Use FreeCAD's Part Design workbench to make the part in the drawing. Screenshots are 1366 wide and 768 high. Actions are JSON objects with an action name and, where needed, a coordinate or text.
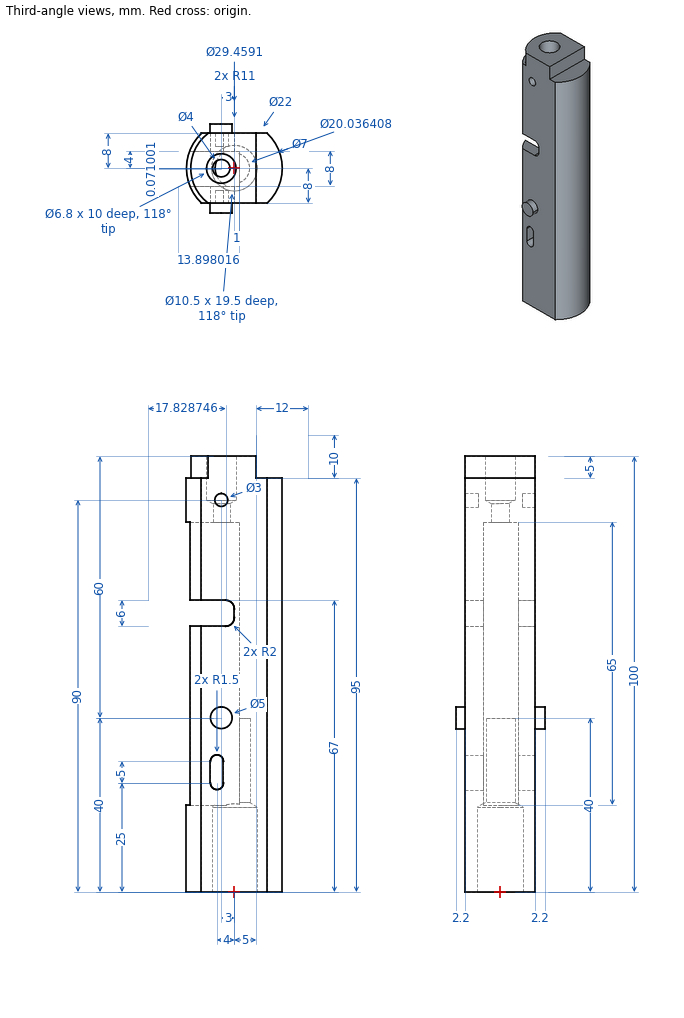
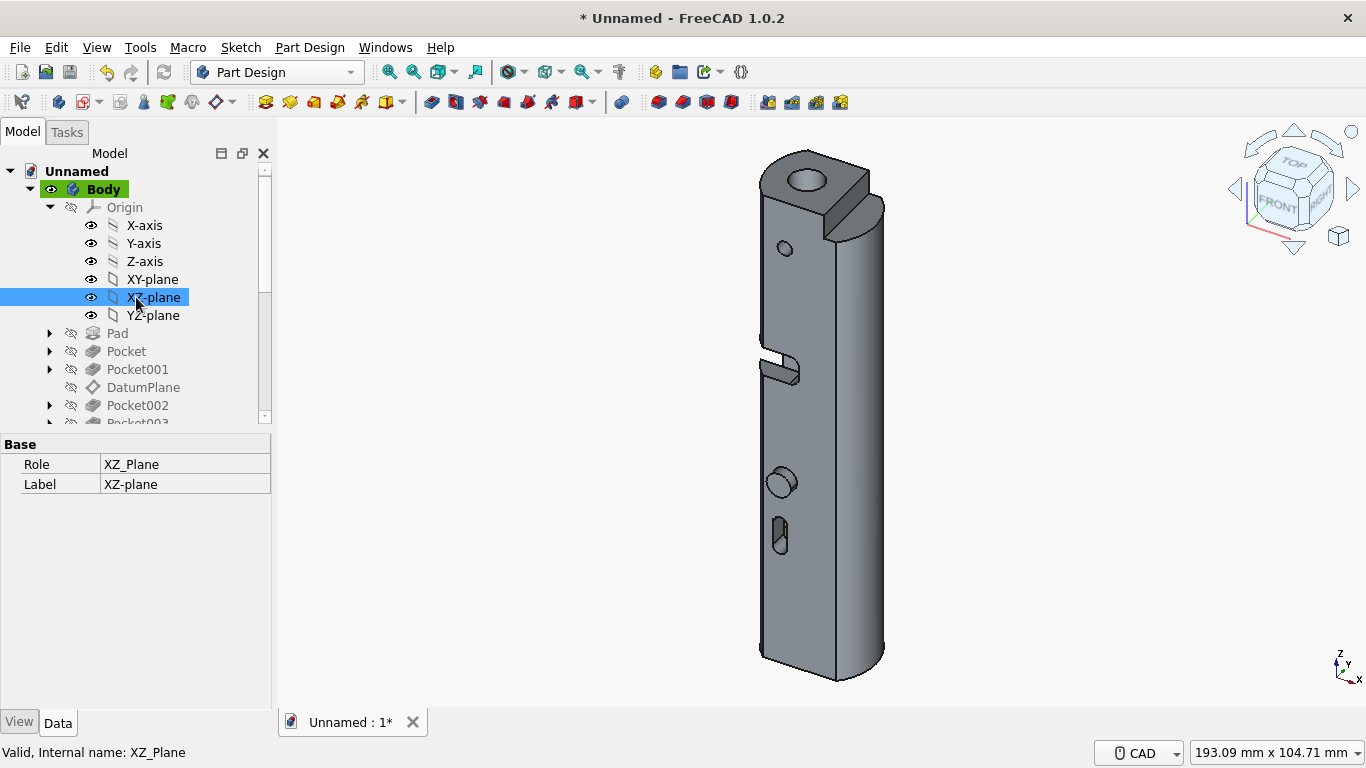
{"action": "left_click", "coordinate": [216, 102]}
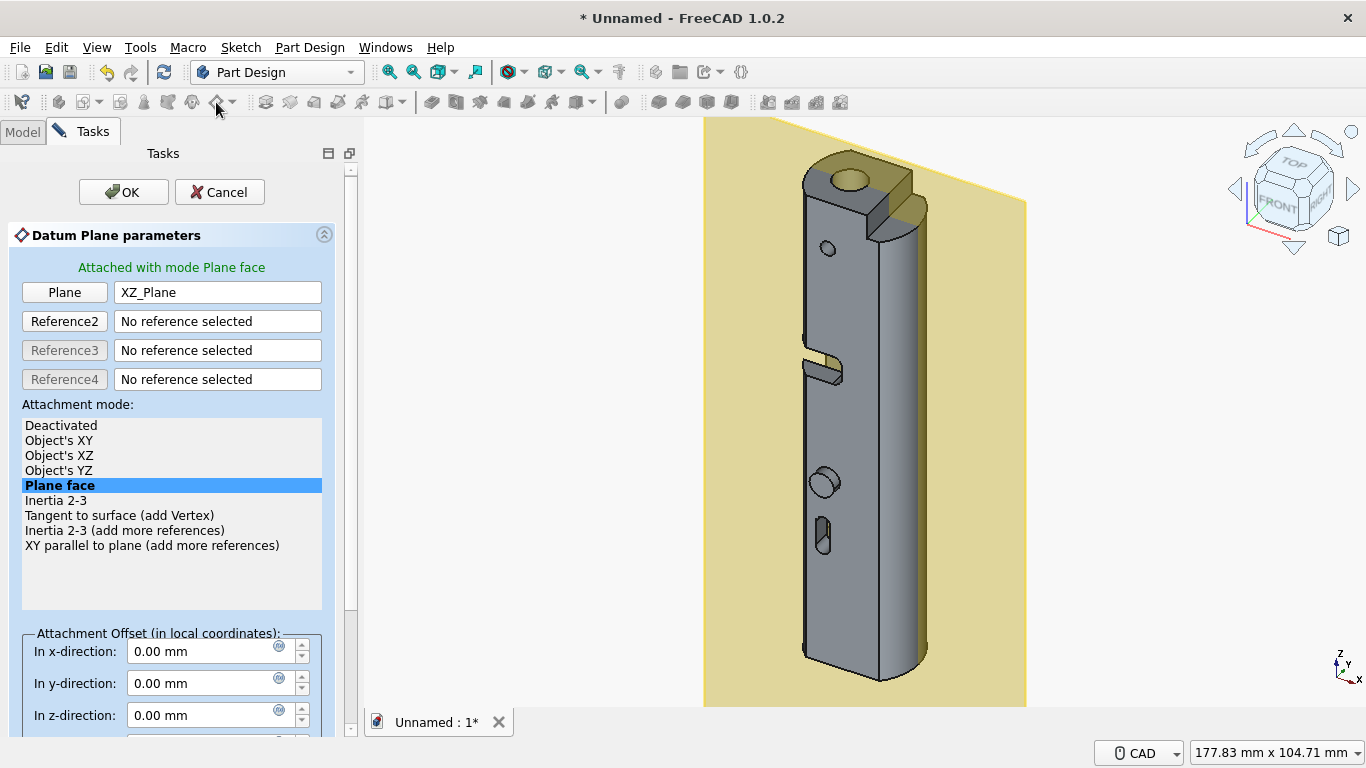
{"action": "triple_click", "coordinate": [210, 715]}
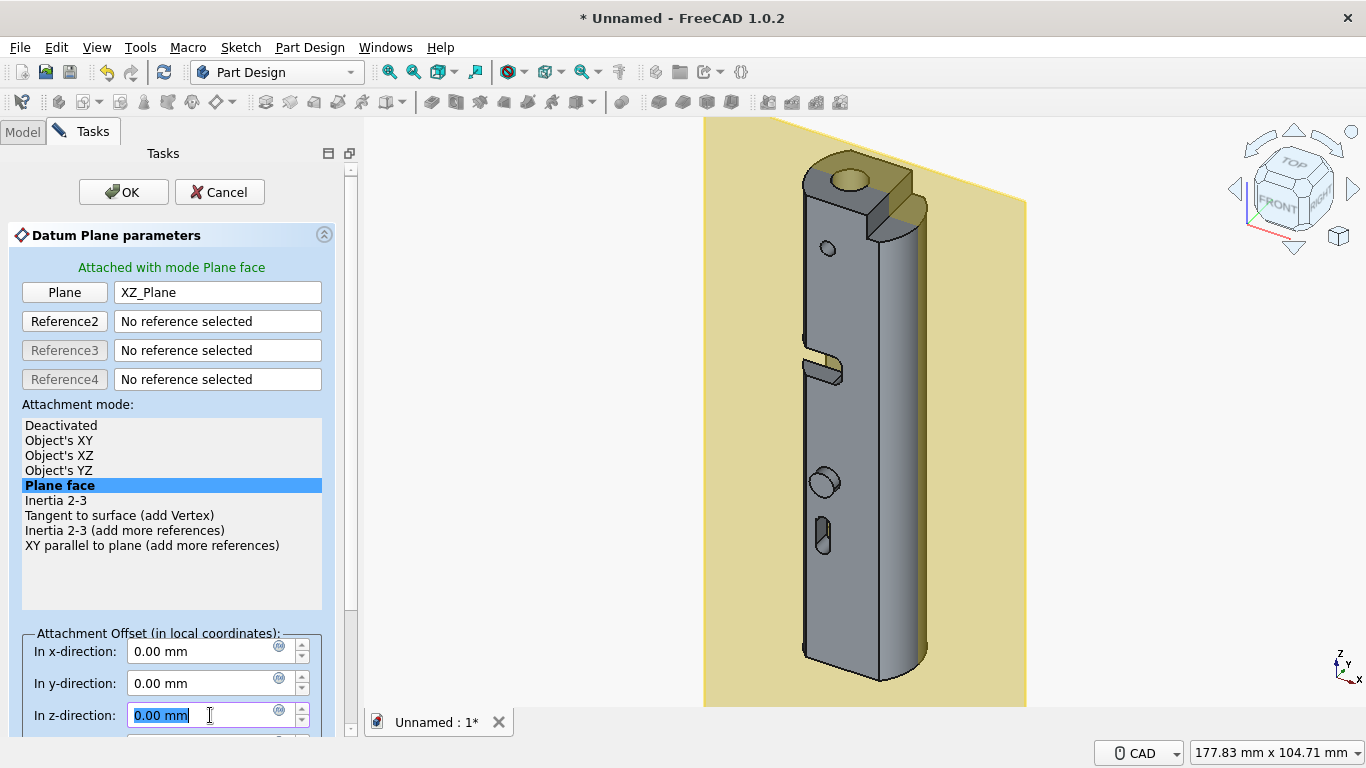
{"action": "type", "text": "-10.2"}
{"action": "key", "text": "Tab"}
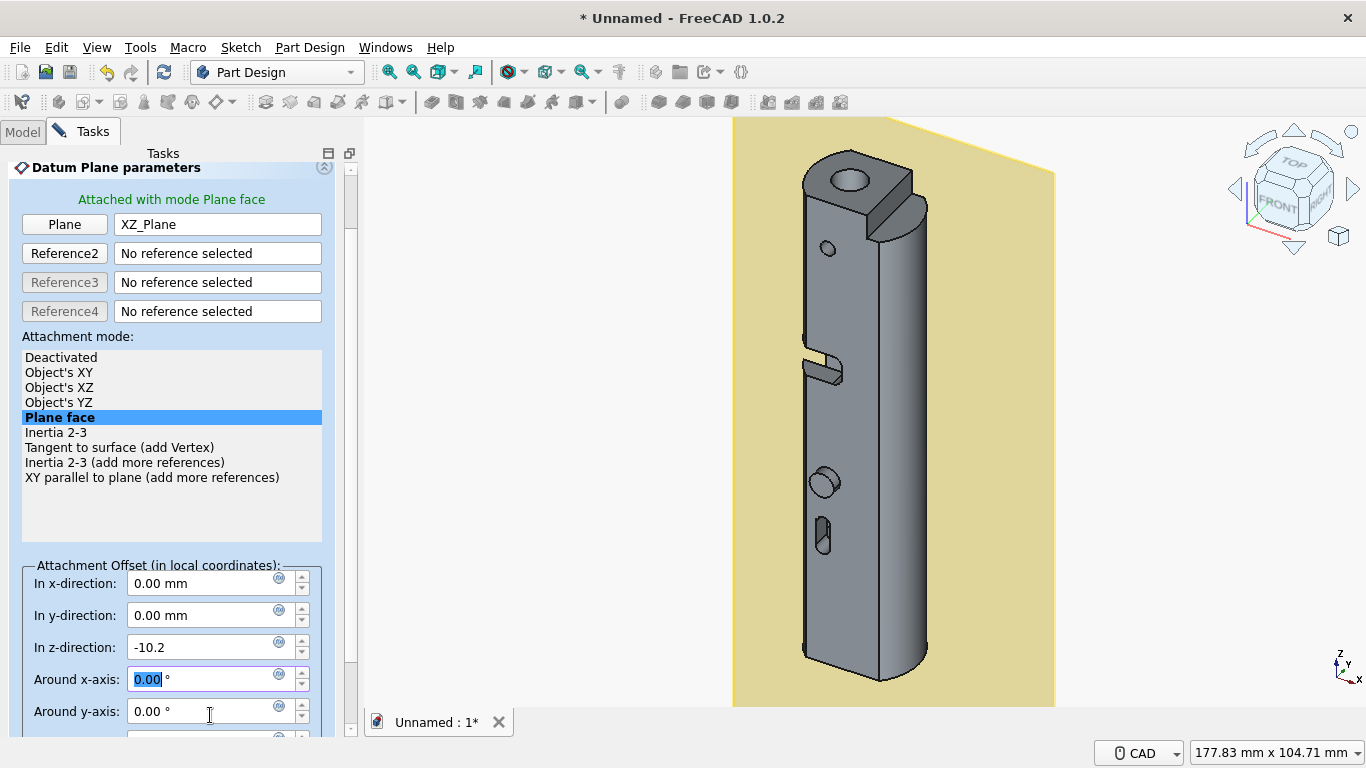
{"action": "scroll", "coordinate": [351, 450], "scroll_direction": "up", "scroll_amount": 2}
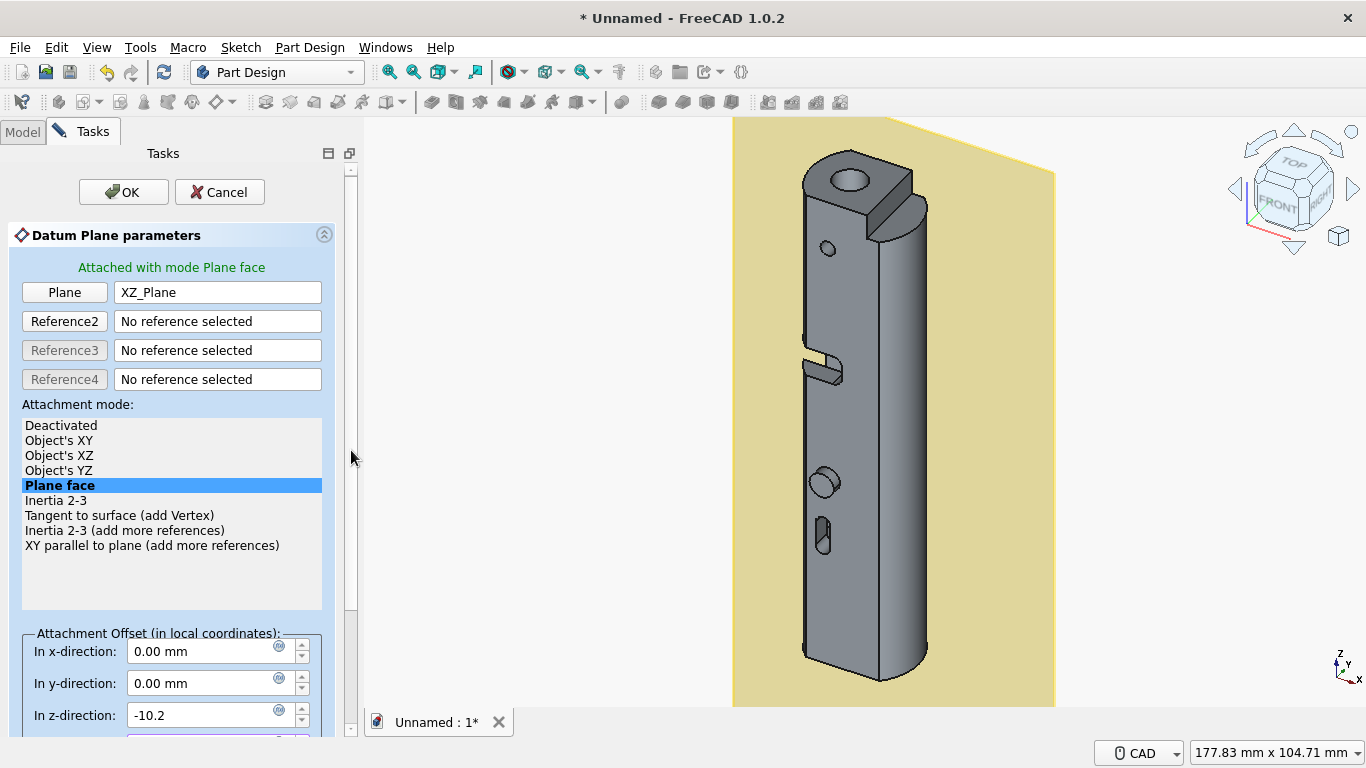
{"action": "left_click", "coordinate": [124, 192]}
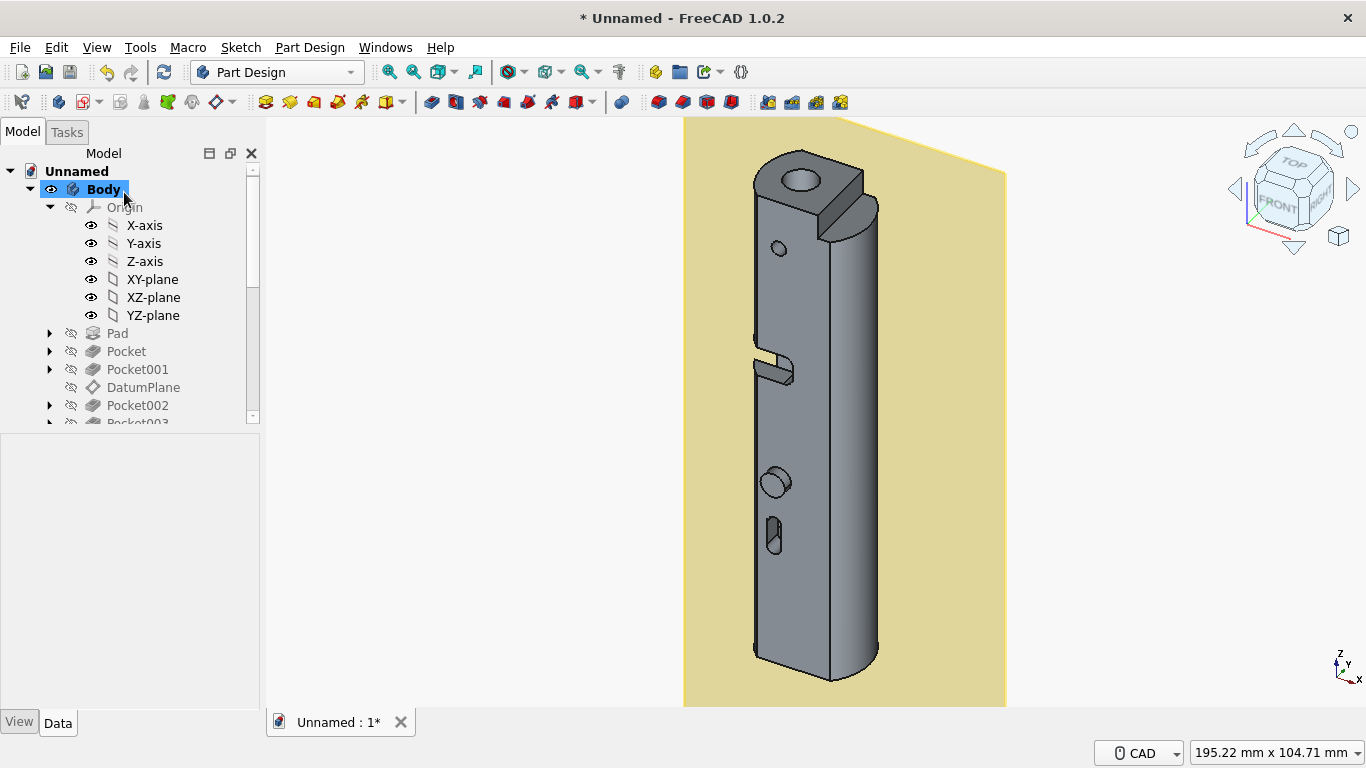
{"action": "scroll", "coordinate": [100, 293], "scroll_direction": "down", "scroll_amount": 3}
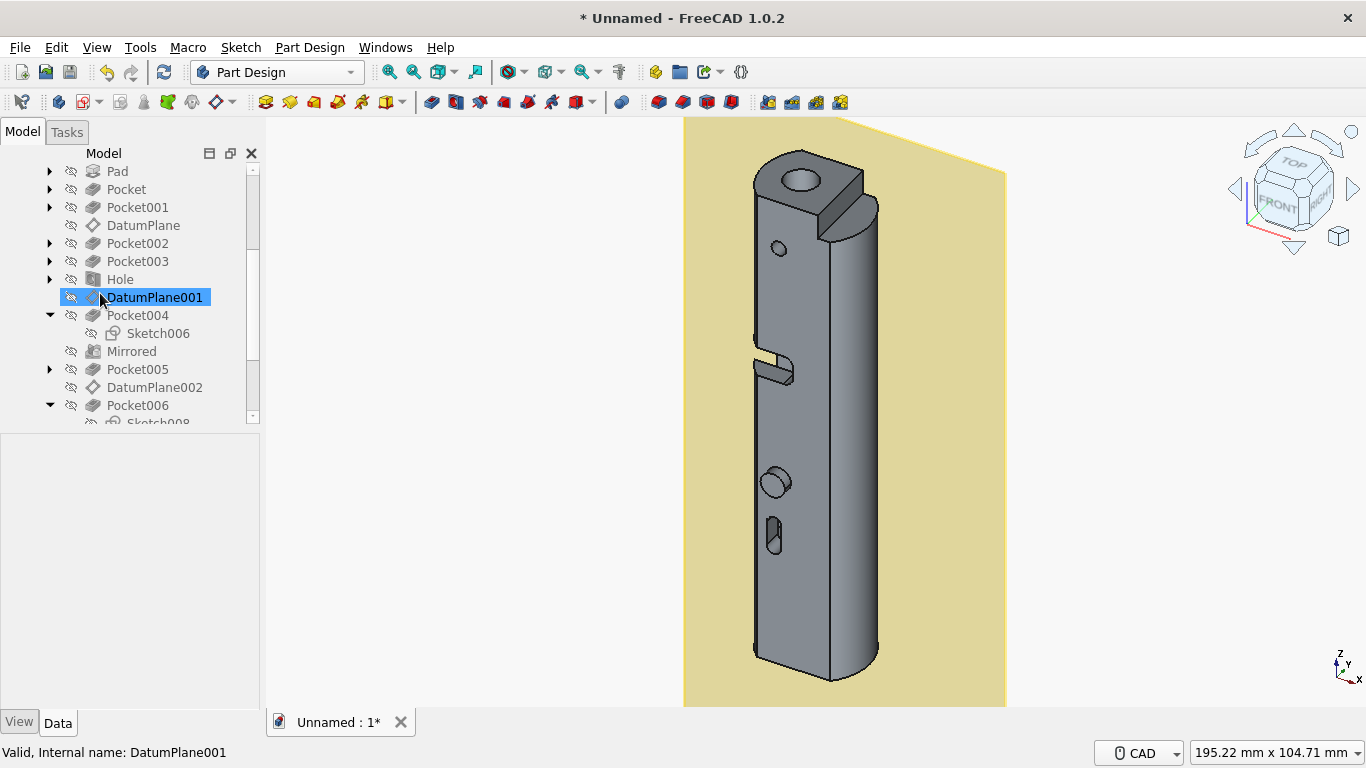
{"action": "scroll", "coordinate": [140, 293], "scroll_direction": "up", "scroll_amount": 15}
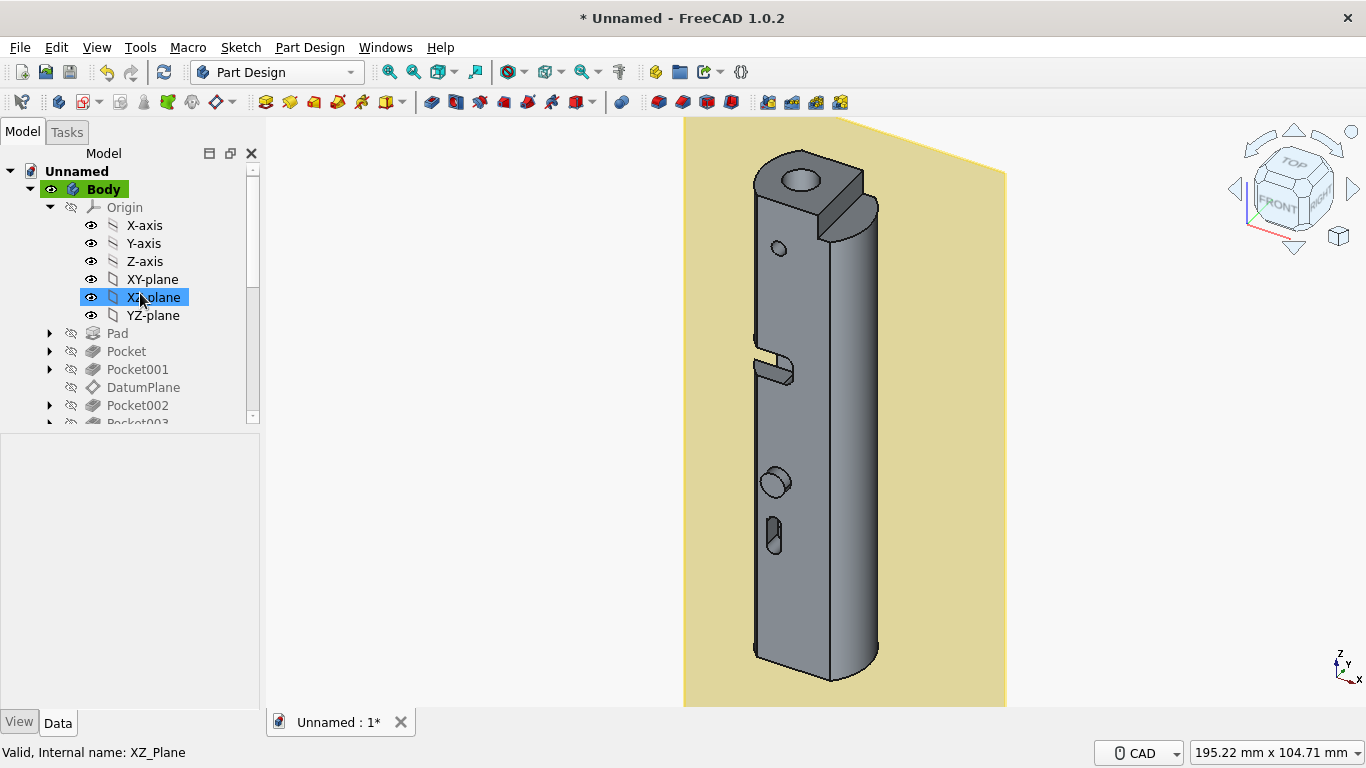
{"action": "scroll", "coordinate": [100, 293], "scroll_direction": "down", "scroll_amount": 6}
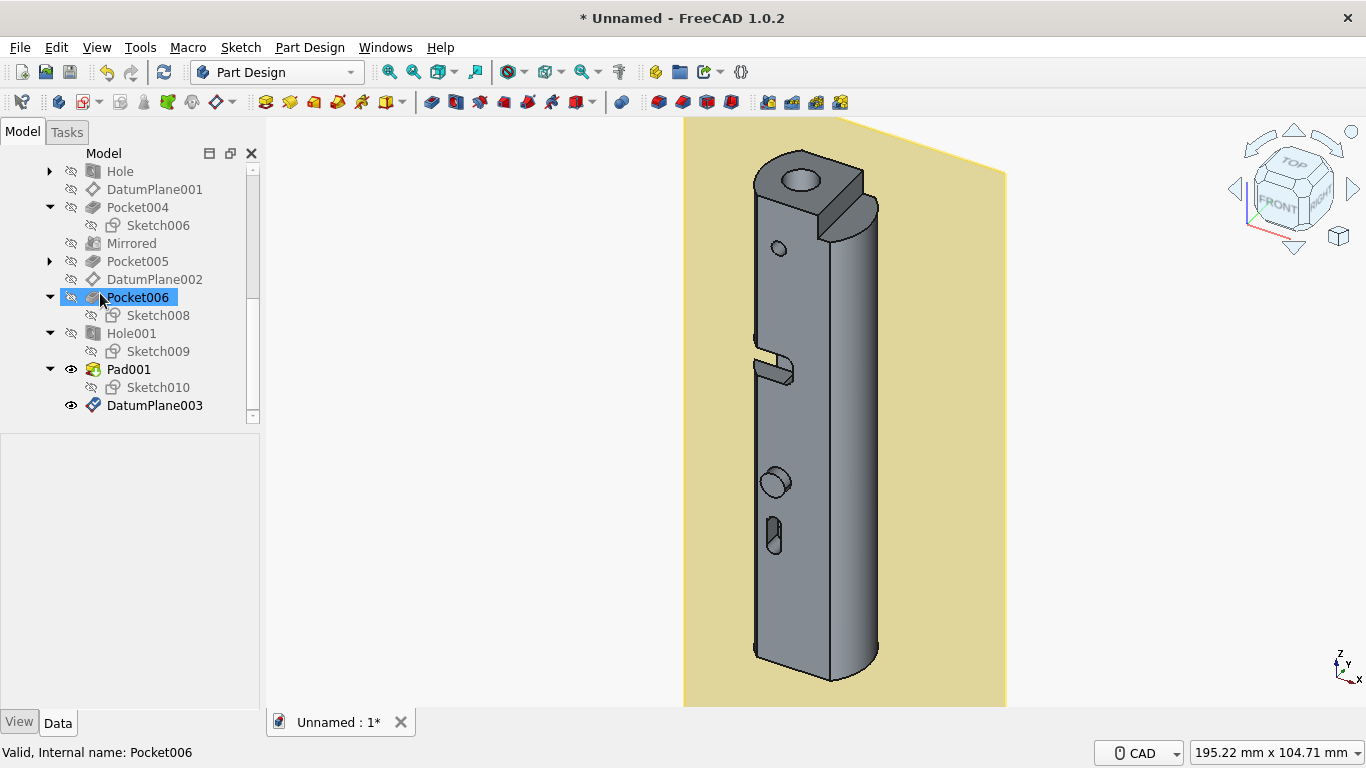
{"action": "left_click", "coordinate": [116, 405]}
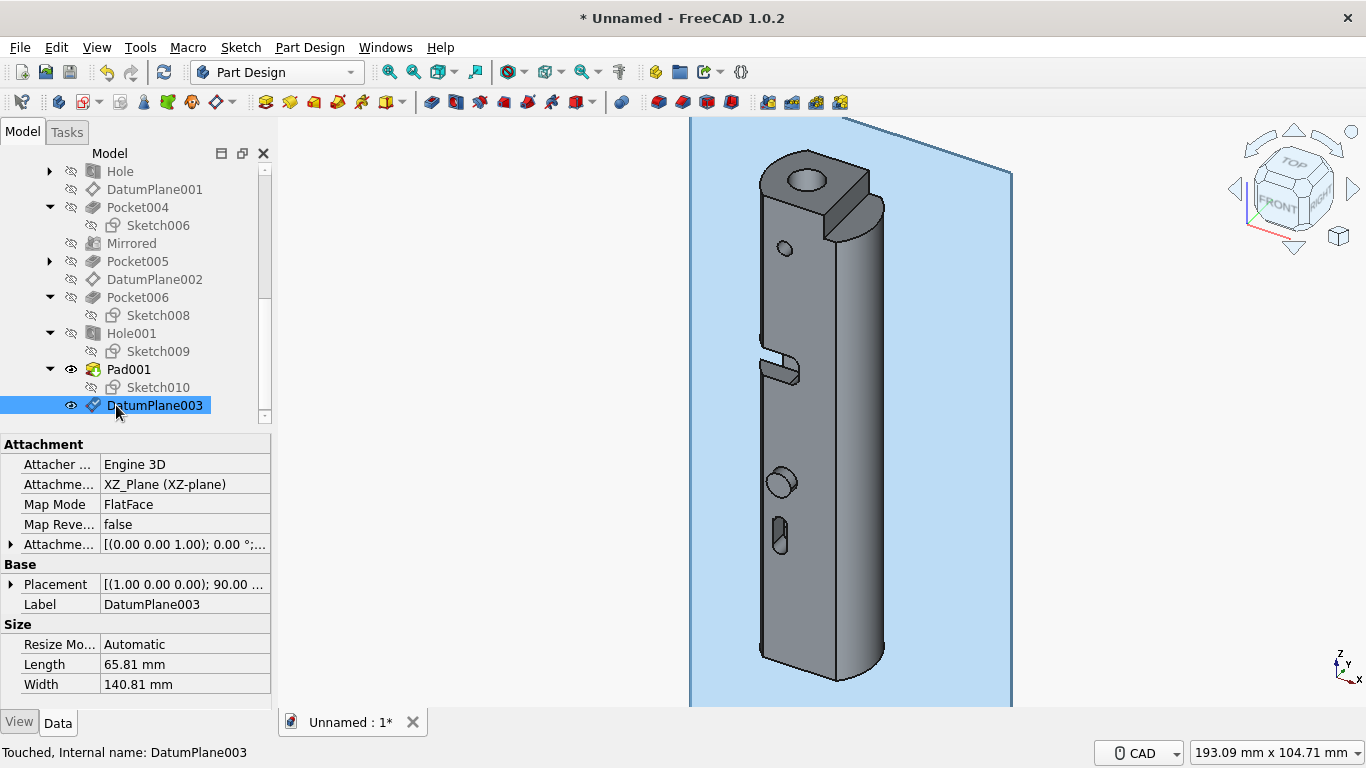
{"action": "left_click", "coordinate": [84, 102]}